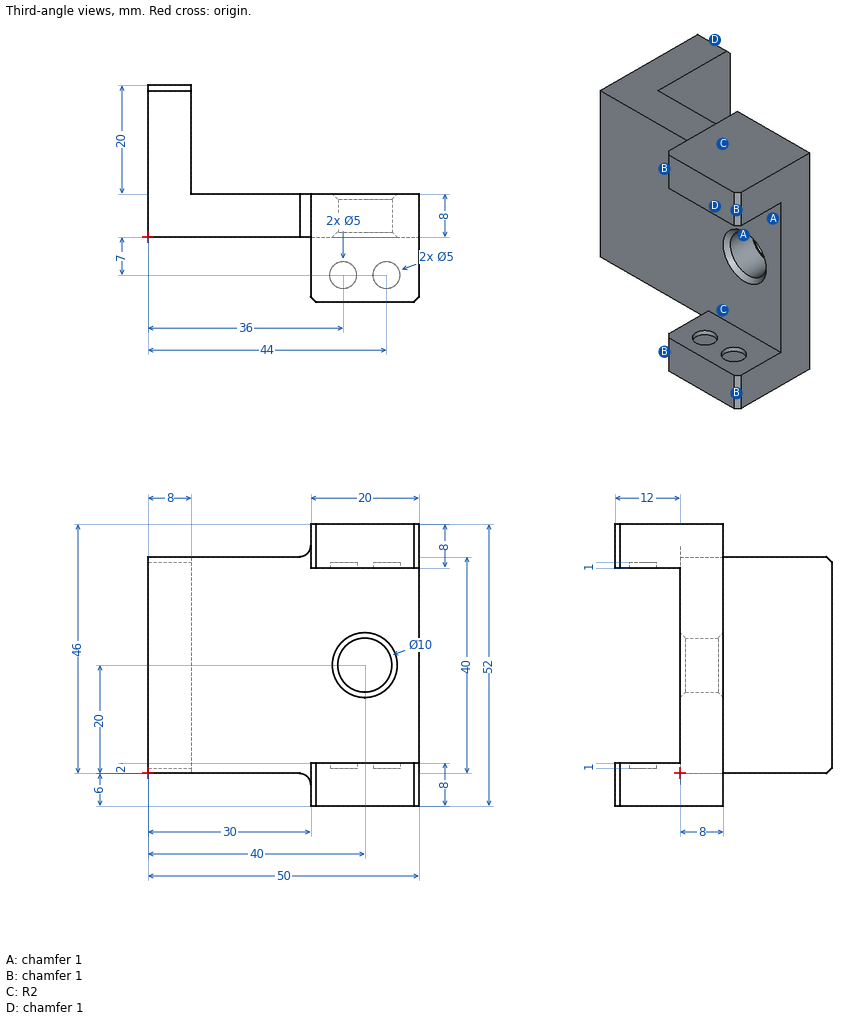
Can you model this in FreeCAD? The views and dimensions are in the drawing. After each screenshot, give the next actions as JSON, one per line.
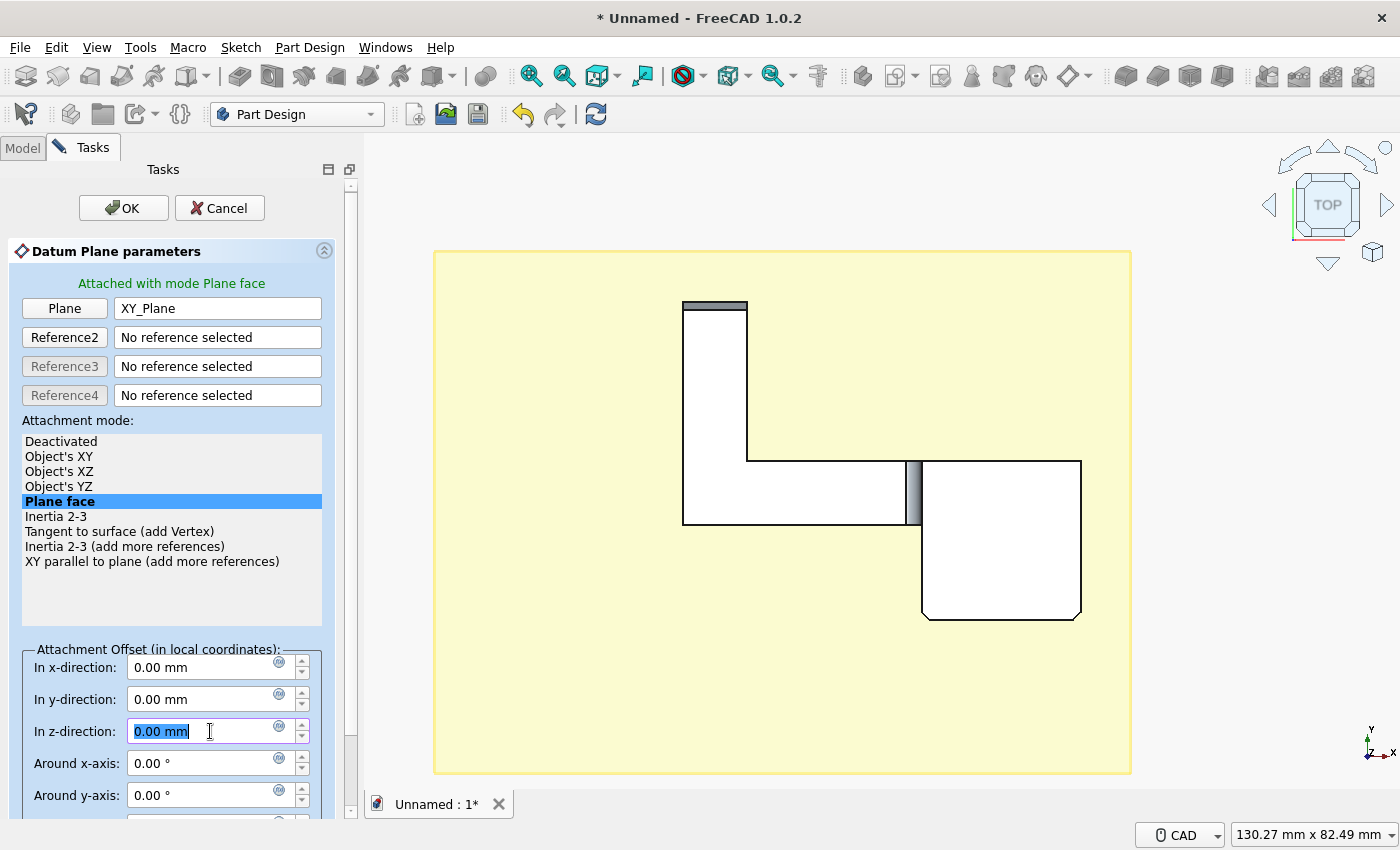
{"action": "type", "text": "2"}
{"action": "key", "text": "Tab"}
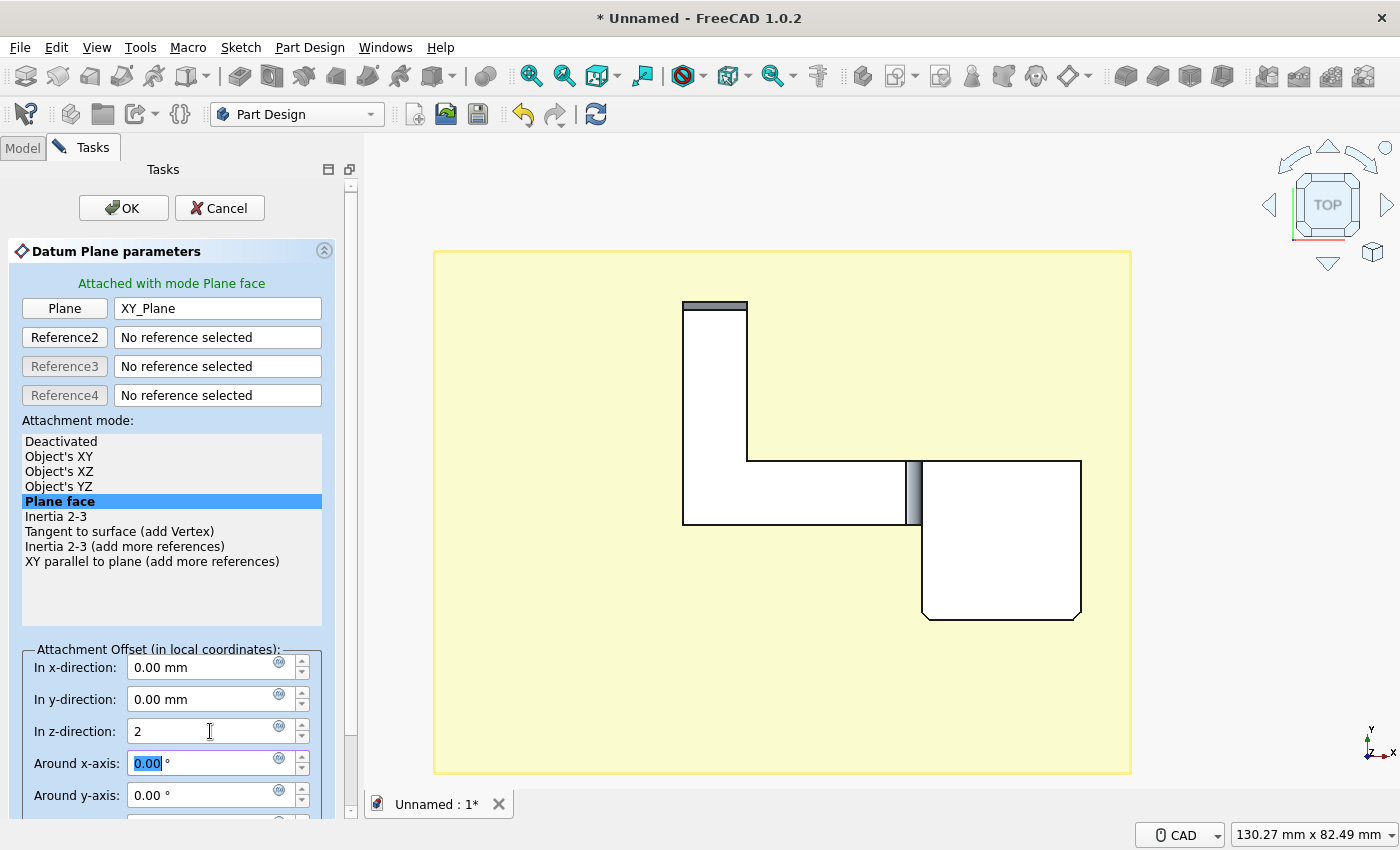
{"action": "left_click", "coordinate": [124, 208]}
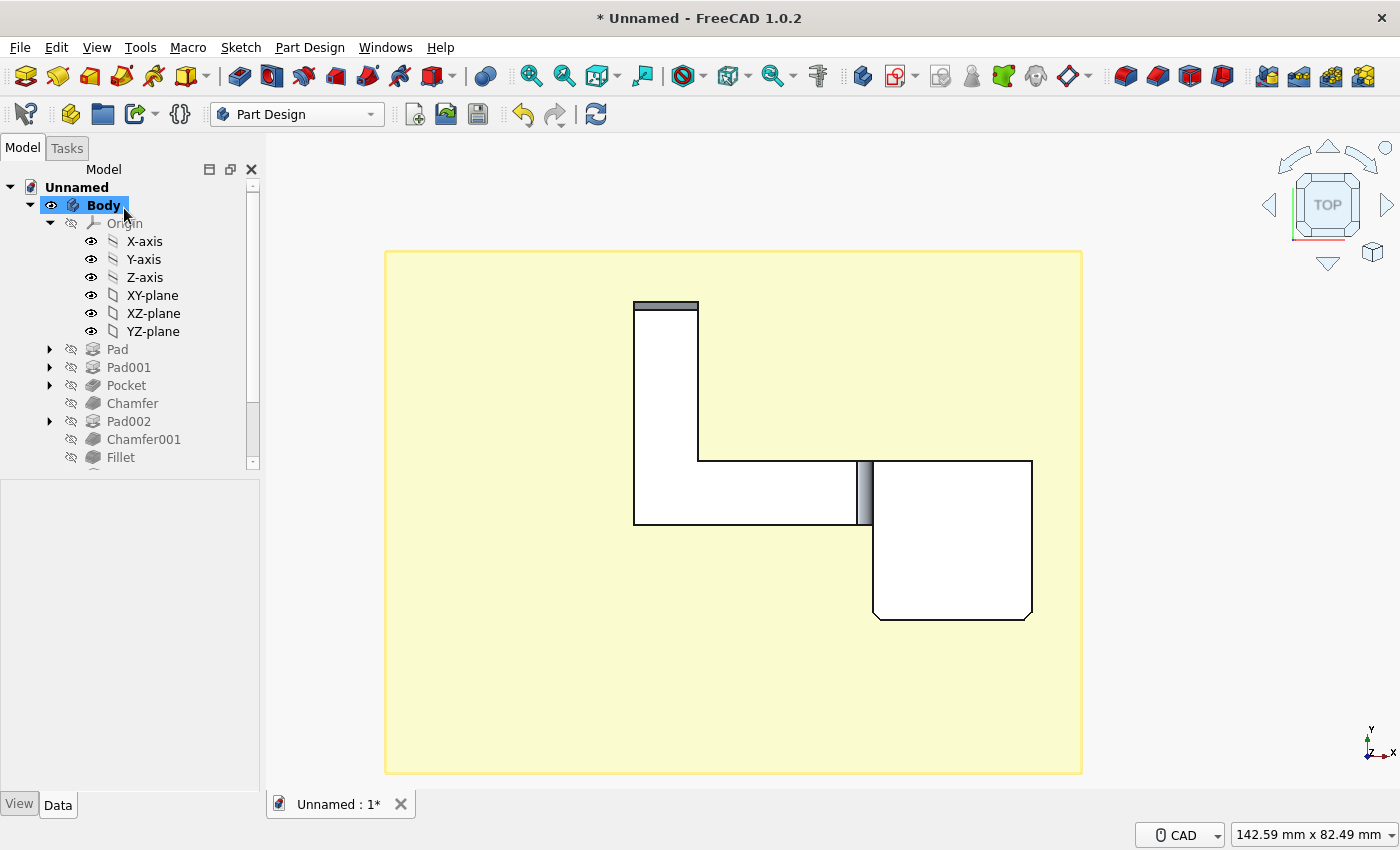
{"action": "scroll", "coordinate": [100, 327], "scroll_direction": "down", "scroll_amount": 3}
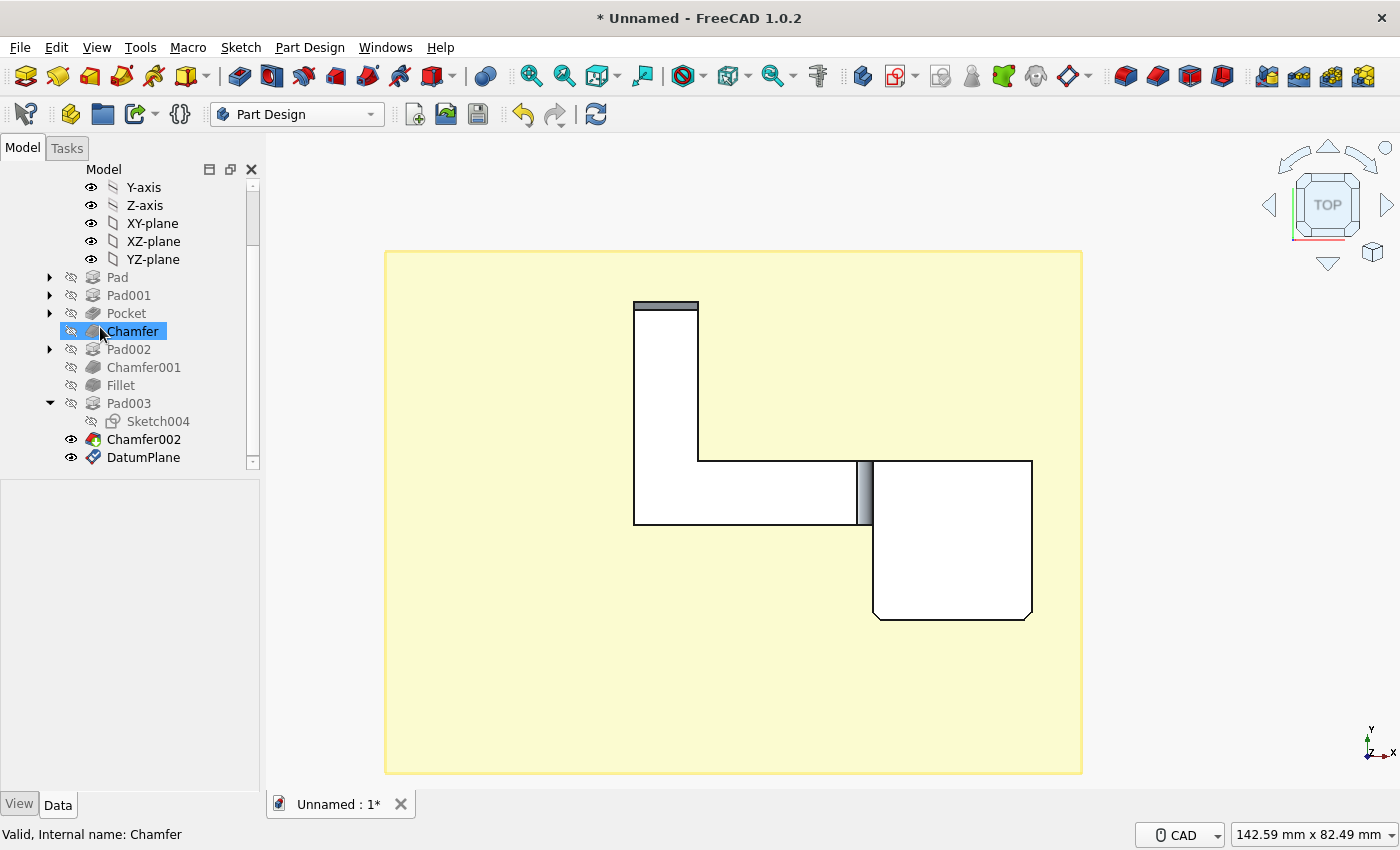
{"action": "left_click", "coordinate": [116, 457]}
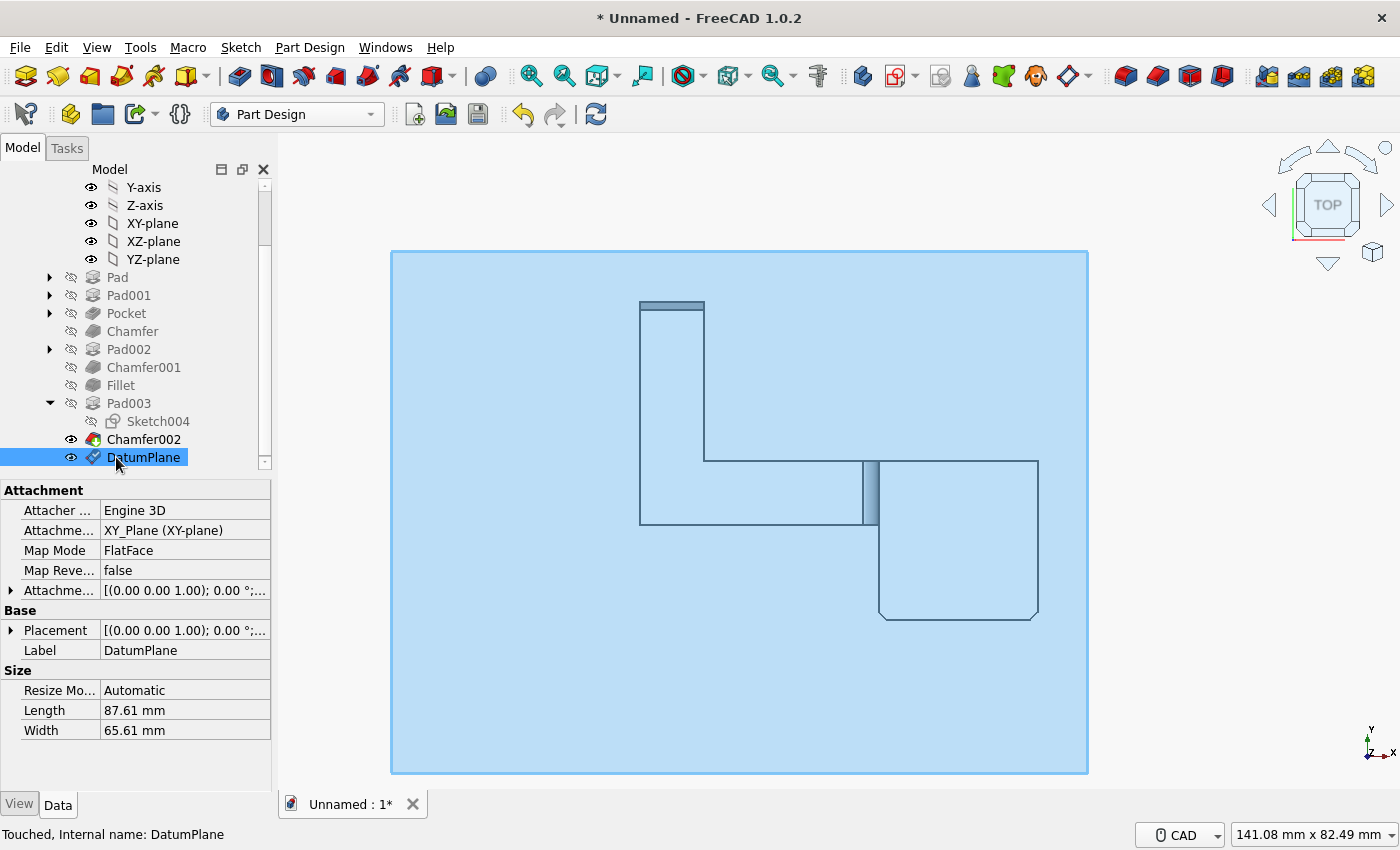
{"action": "left_click", "coordinate": [896, 76]}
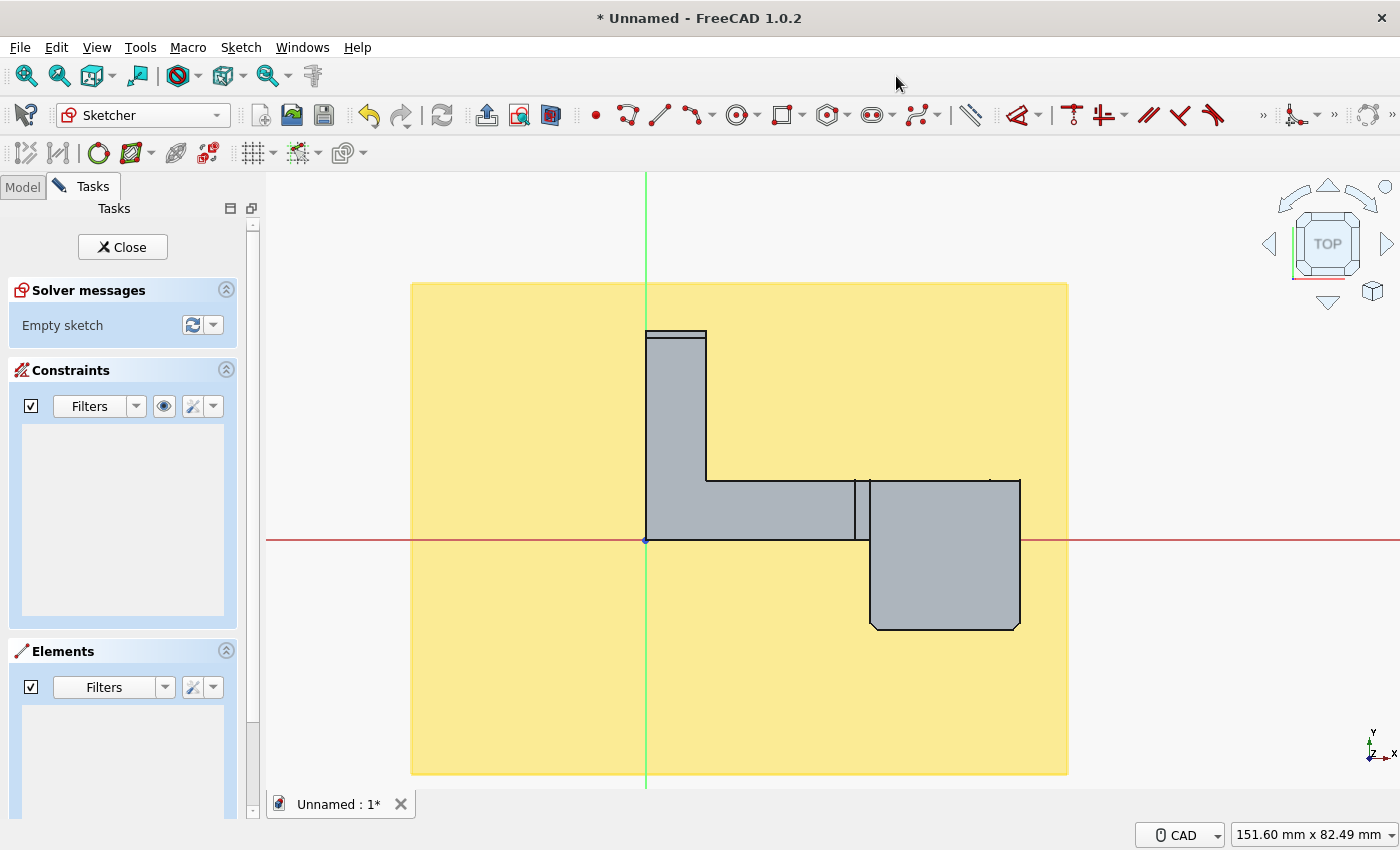
{"action": "left_click", "coordinate": [552, 116]}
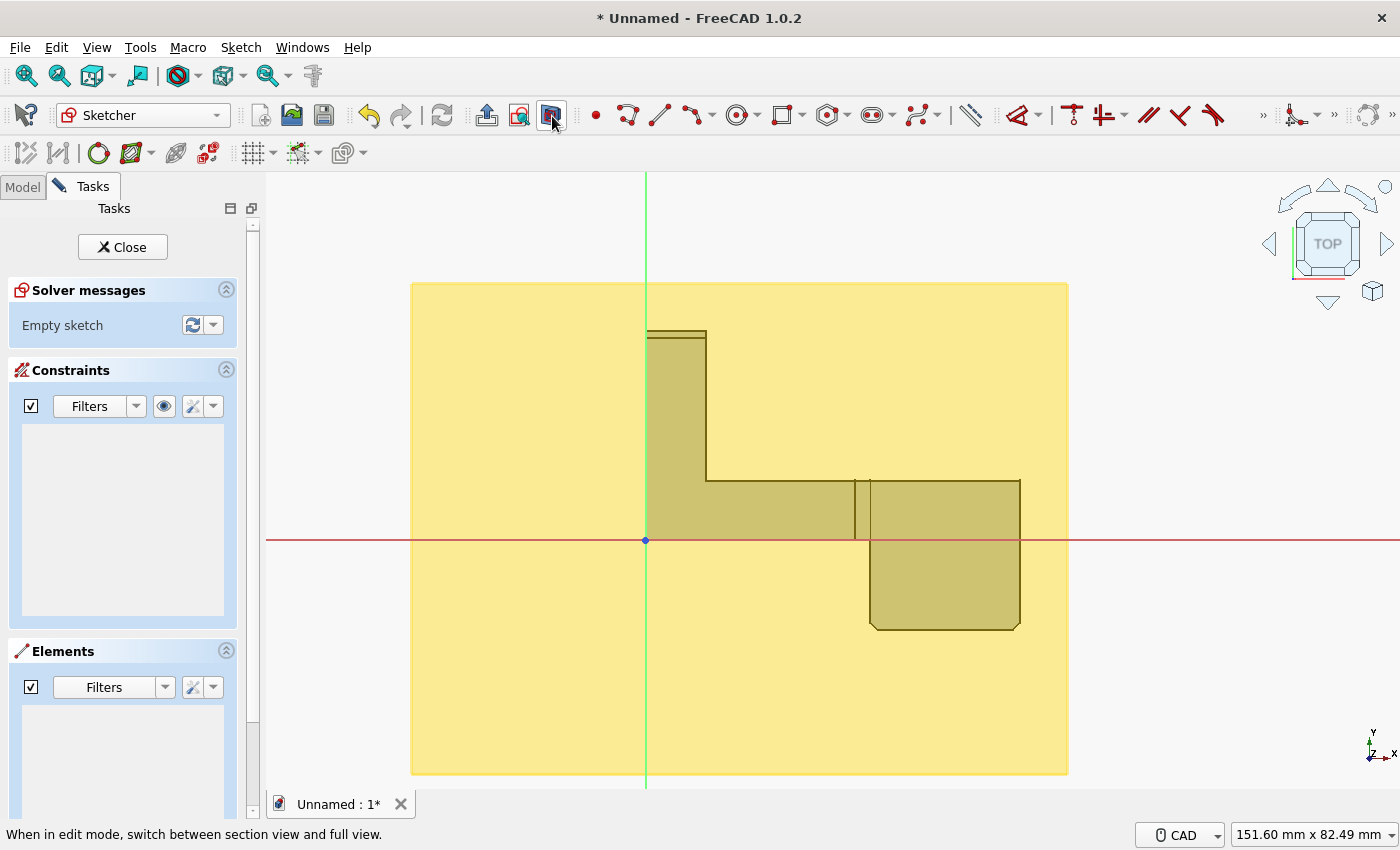
{"action": "scroll", "coordinate": [973, 610], "scroll_direction": "up", "scroll_amount": 10}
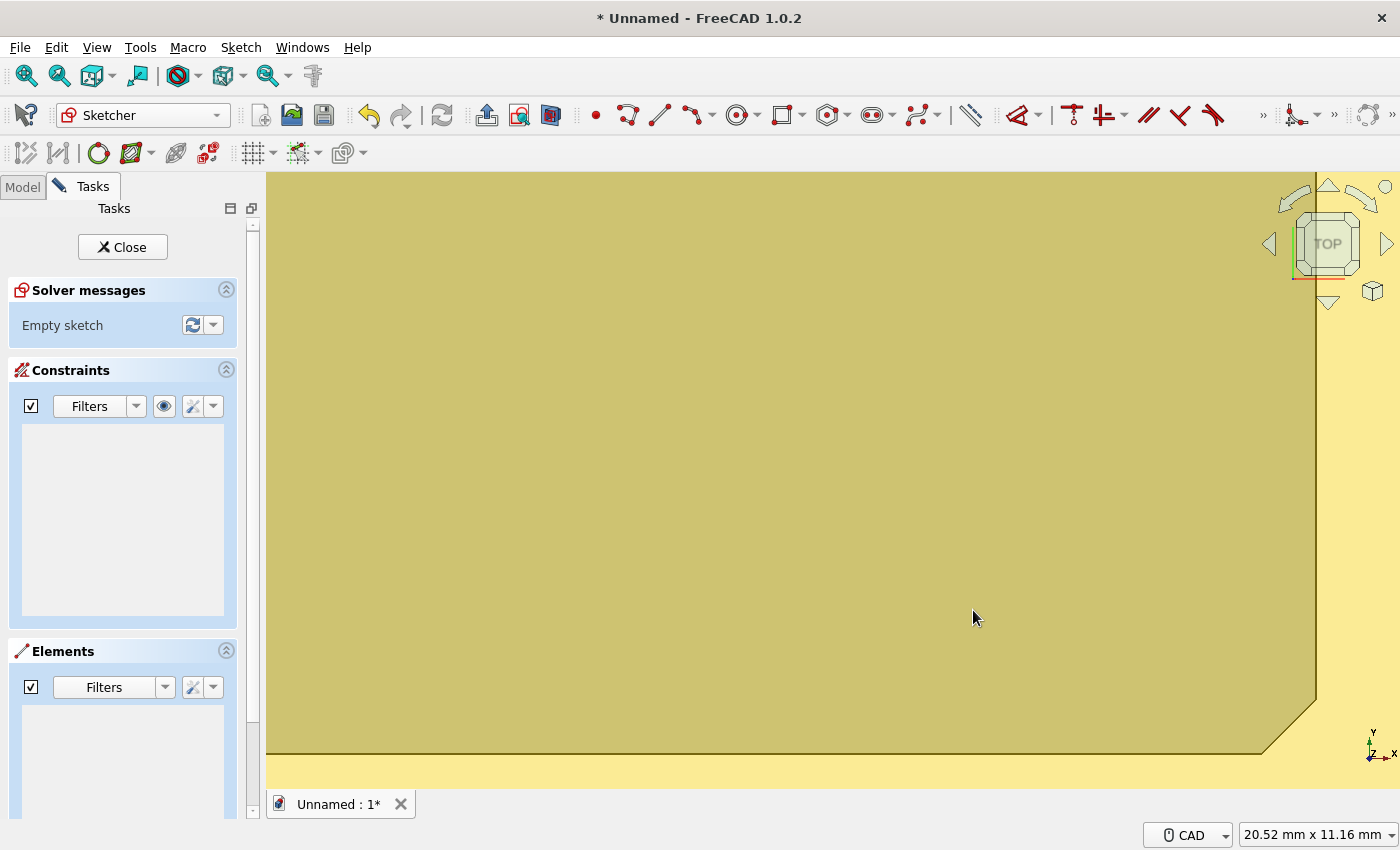
{"action": "left_click", "coordinate": [738, 116]}